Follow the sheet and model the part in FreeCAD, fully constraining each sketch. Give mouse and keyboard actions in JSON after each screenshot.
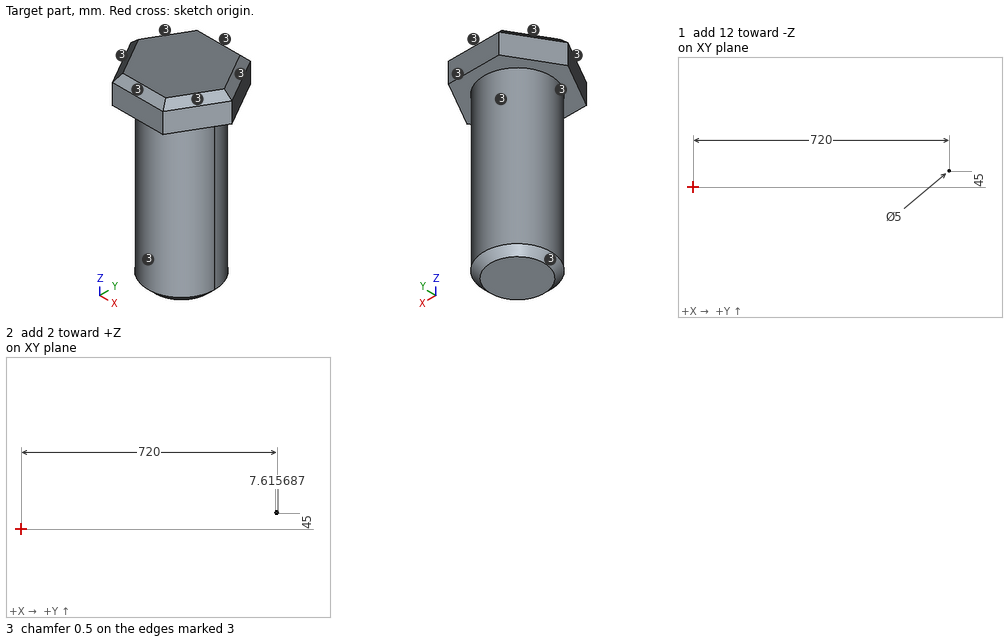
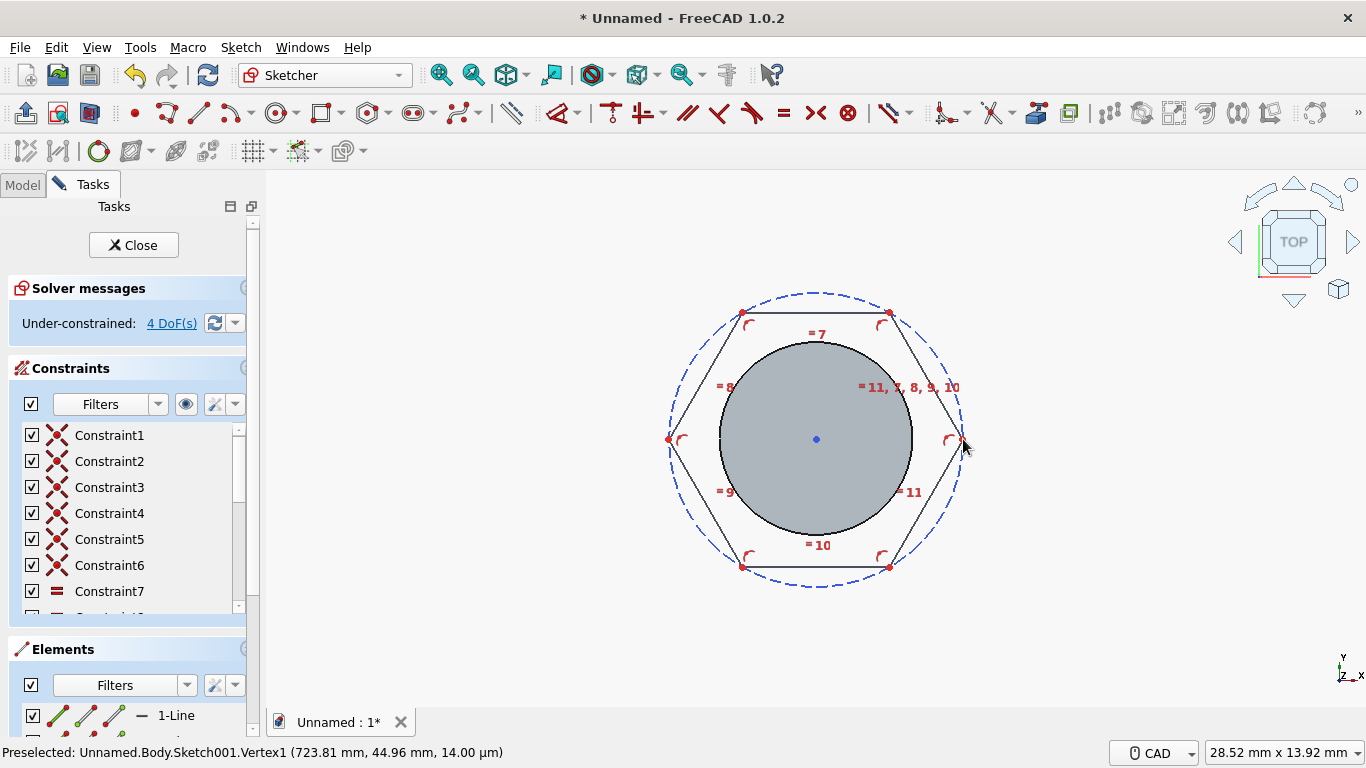
{"action": "left_click", "coordinate": [845, 313]}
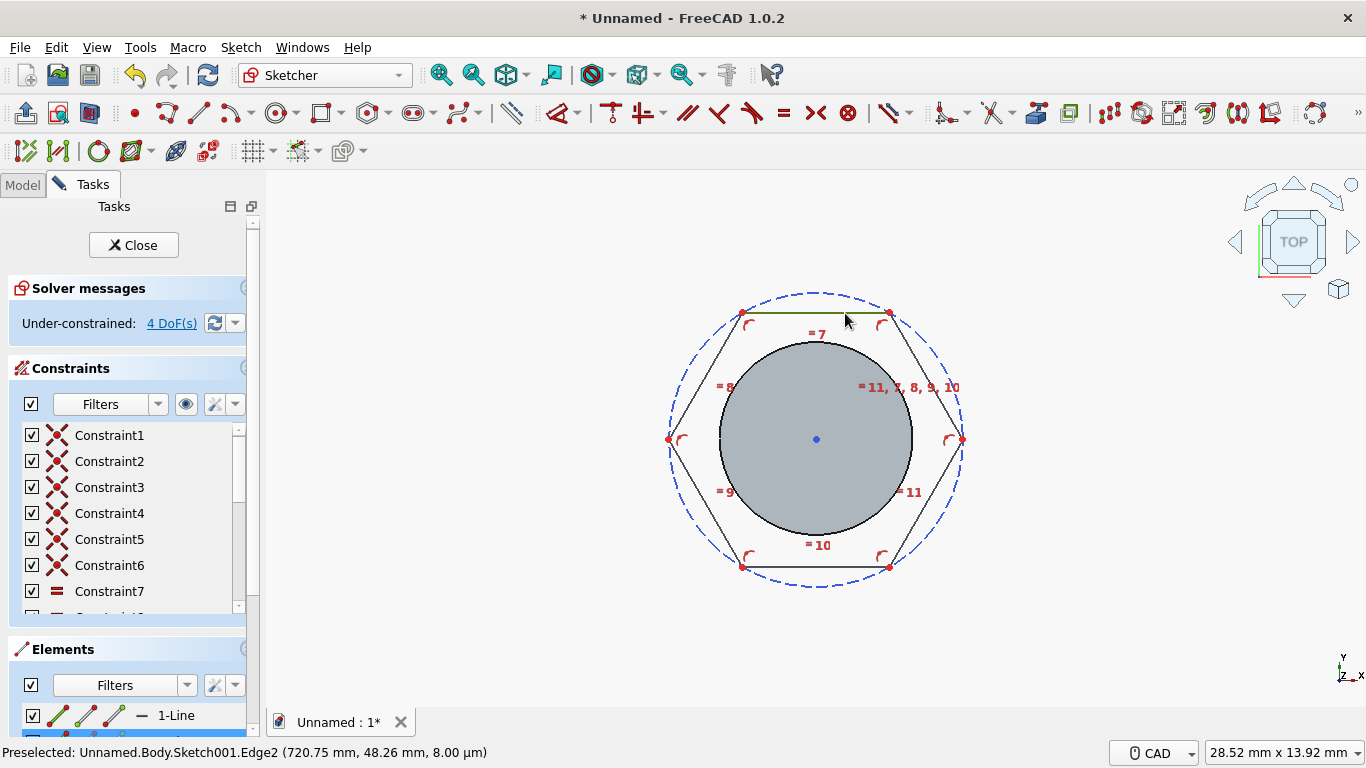
{"action": "key", "text": "h"}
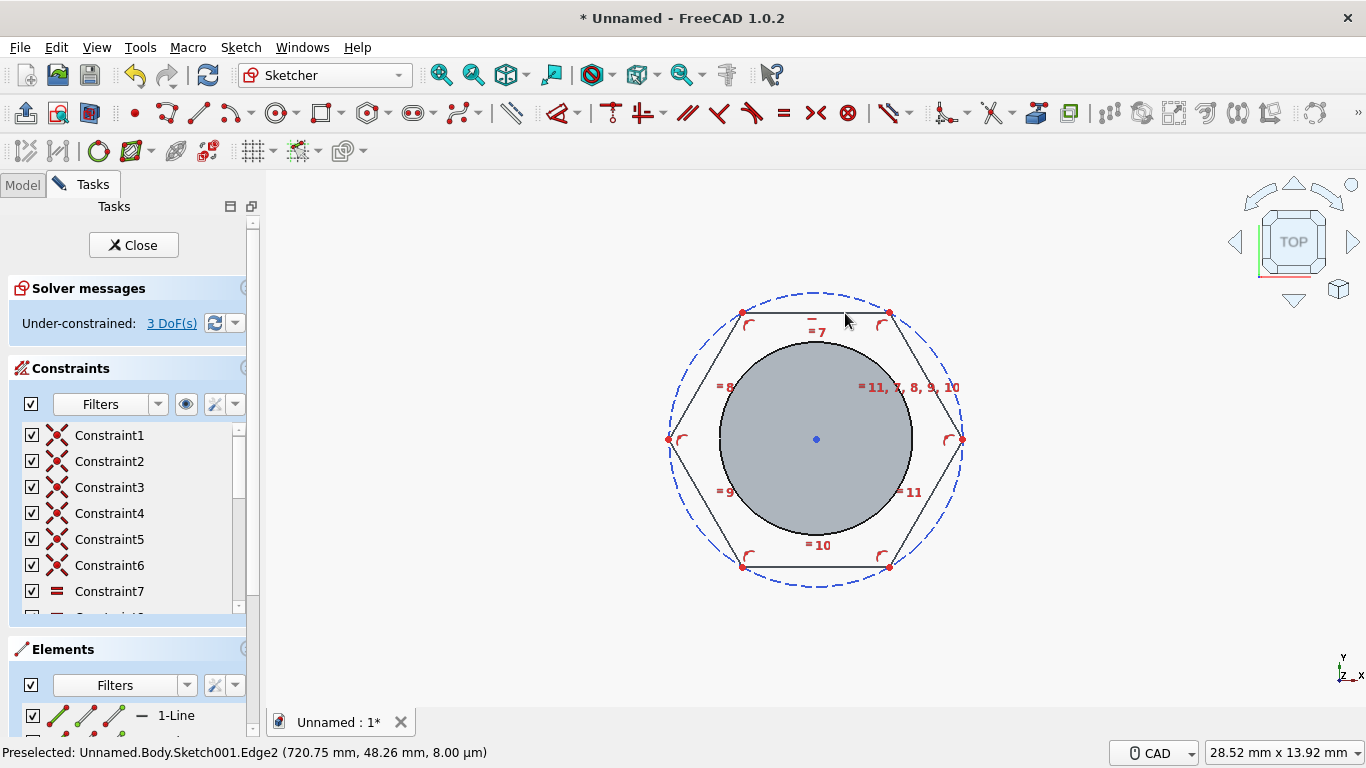
{"action": "left_click", "coordinate": [558, 114]}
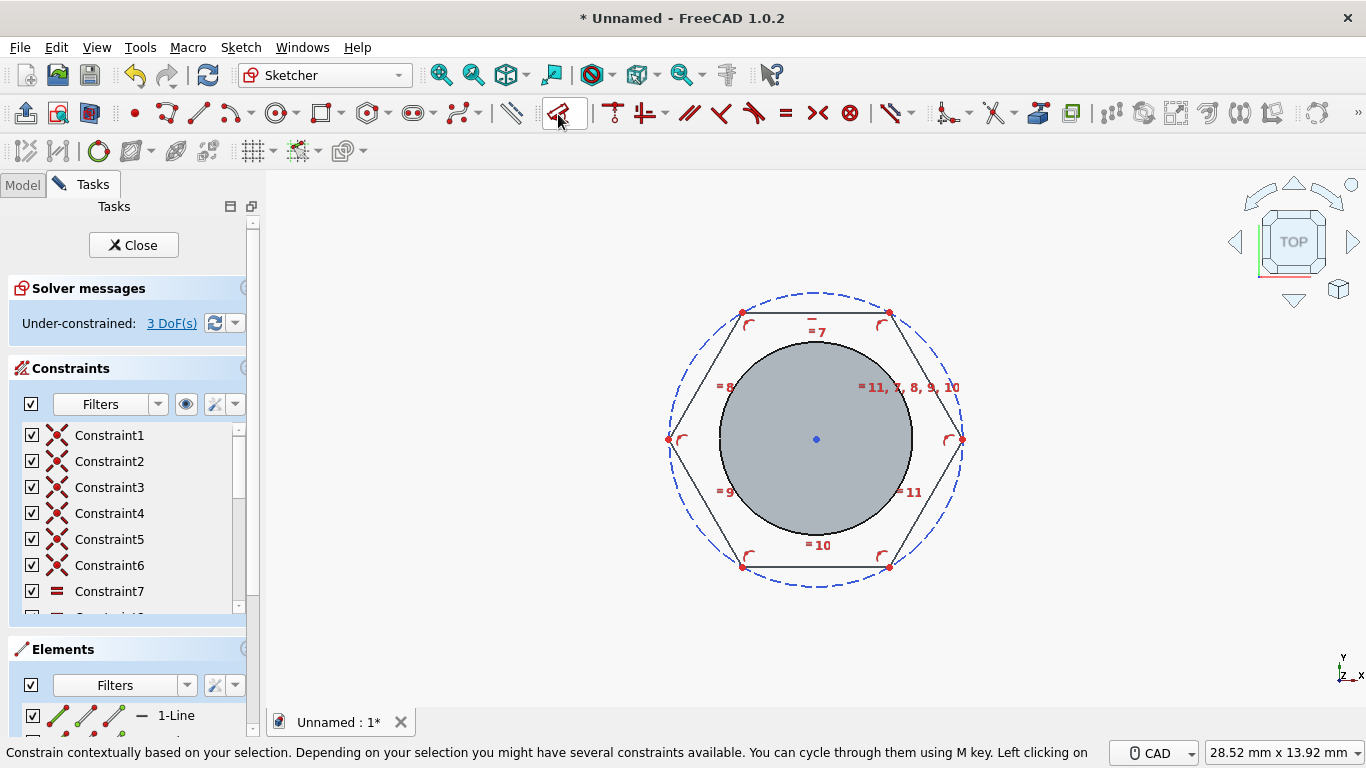
{"action": "left_click", "coordinate": [816, 440]}
{"action": "left_click", "coordinate": [850, 505]}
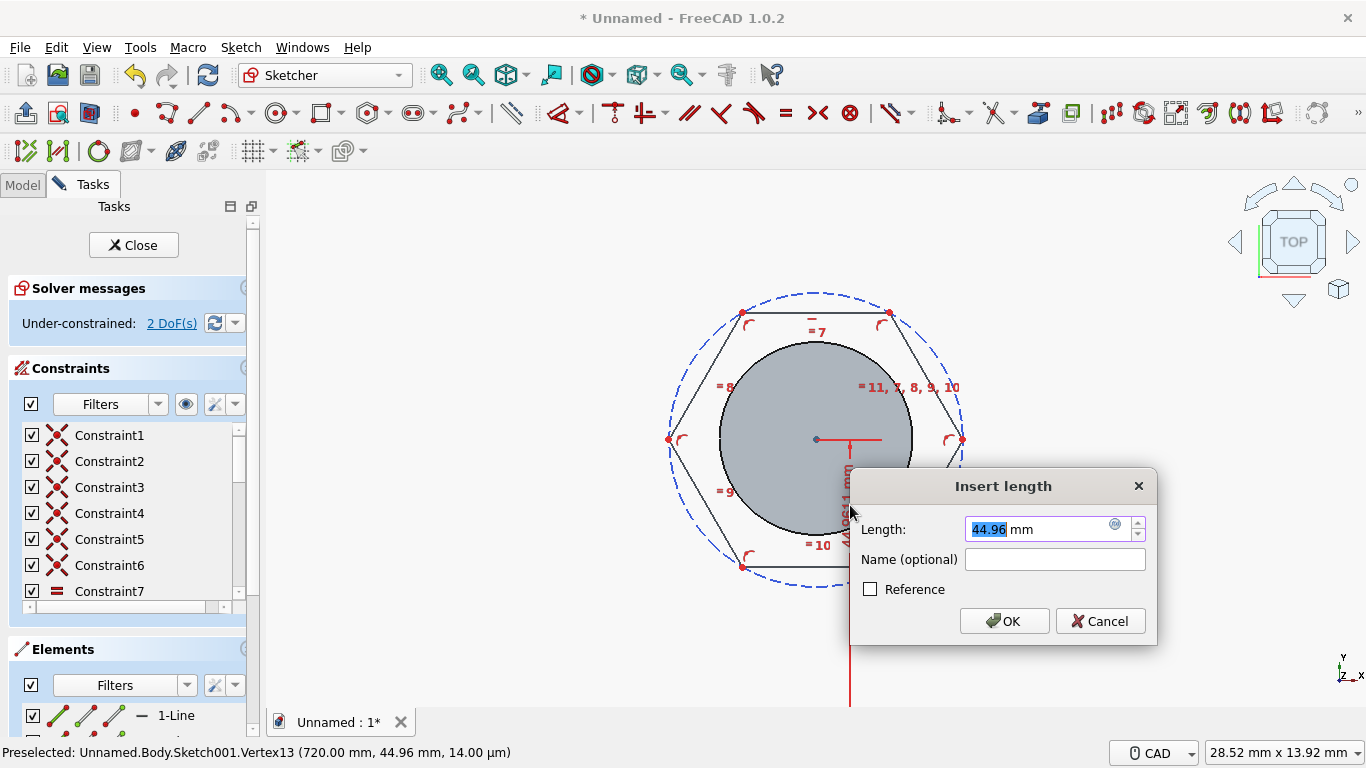
{"action": "type", "text": "45"}
{"action": "key", "text": "Return"}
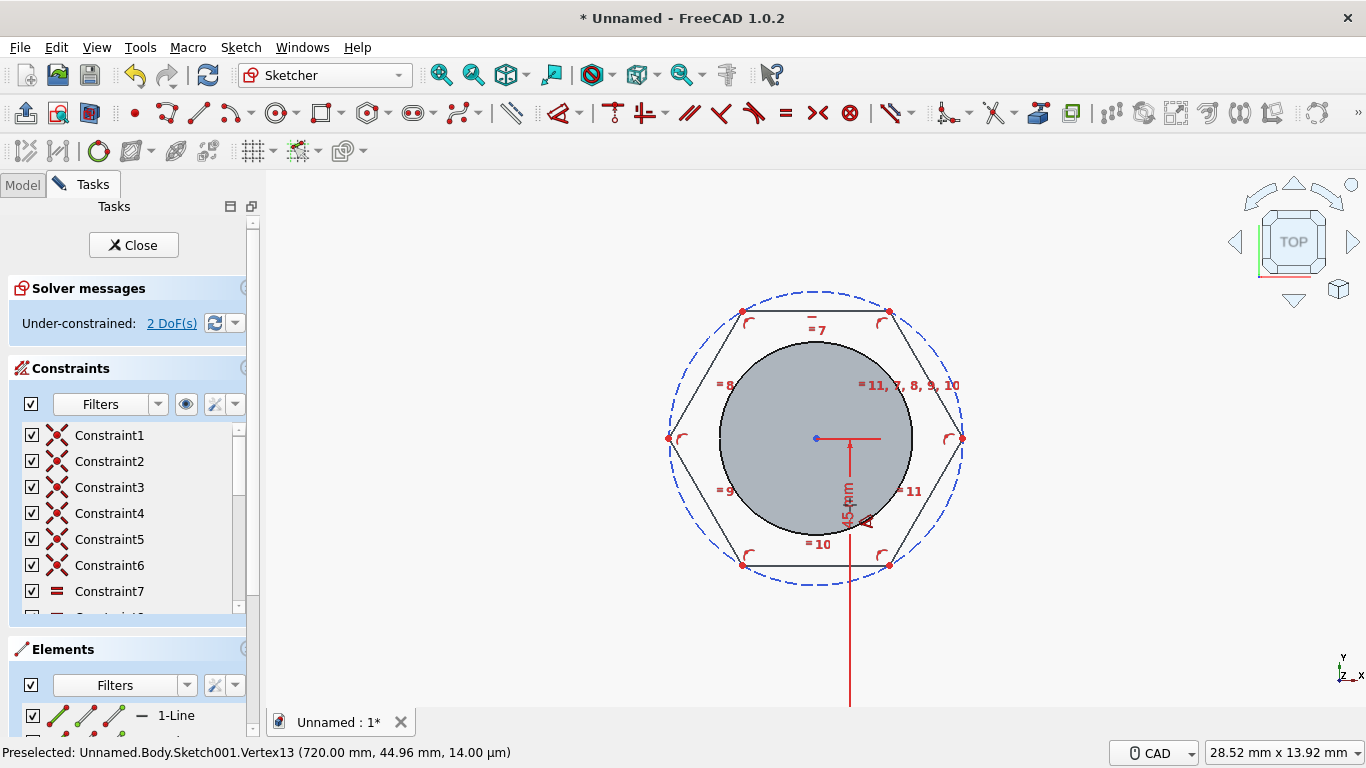
{"action": "left_click", "coordinate": [816, 439]}
{"action": "left_click", "coordinate": [555, 405]}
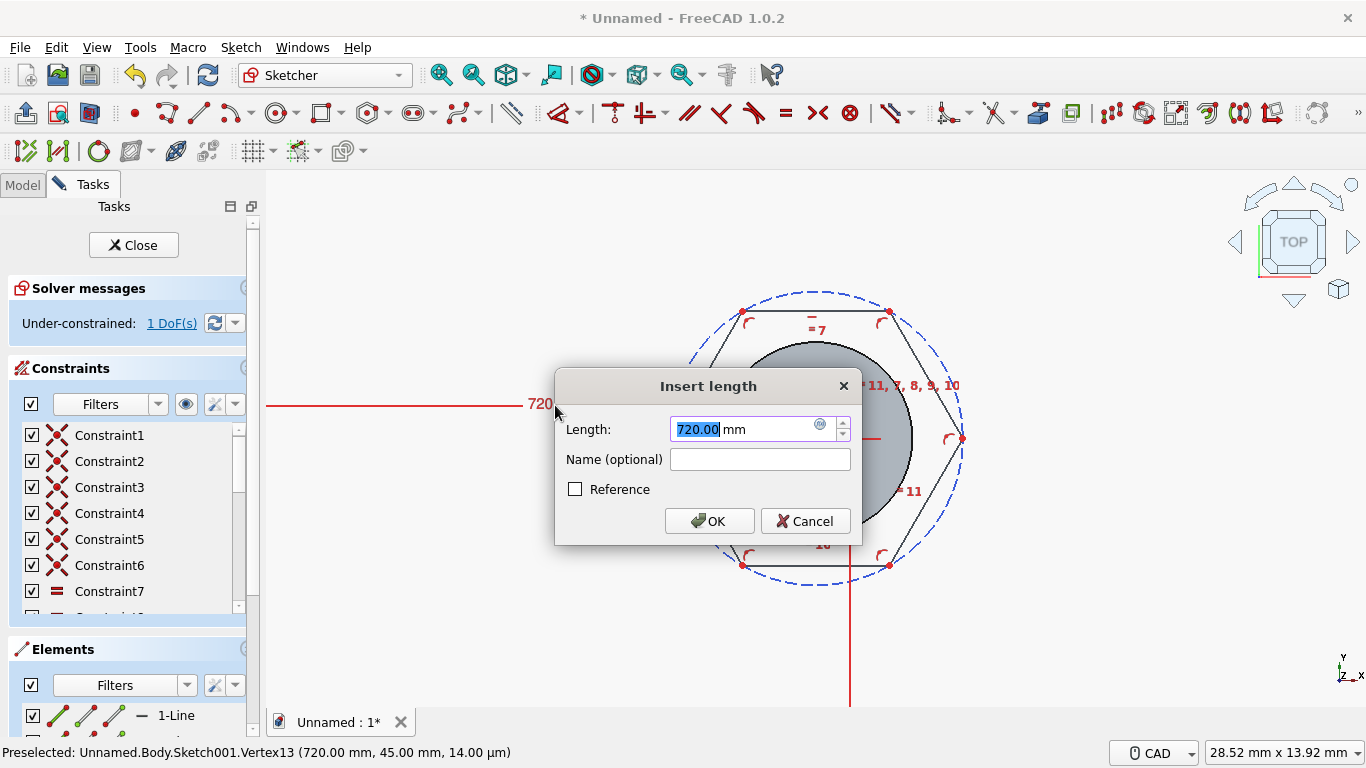
{"action": "type", "text": "720"}
{"action": "key", "text": "Return"}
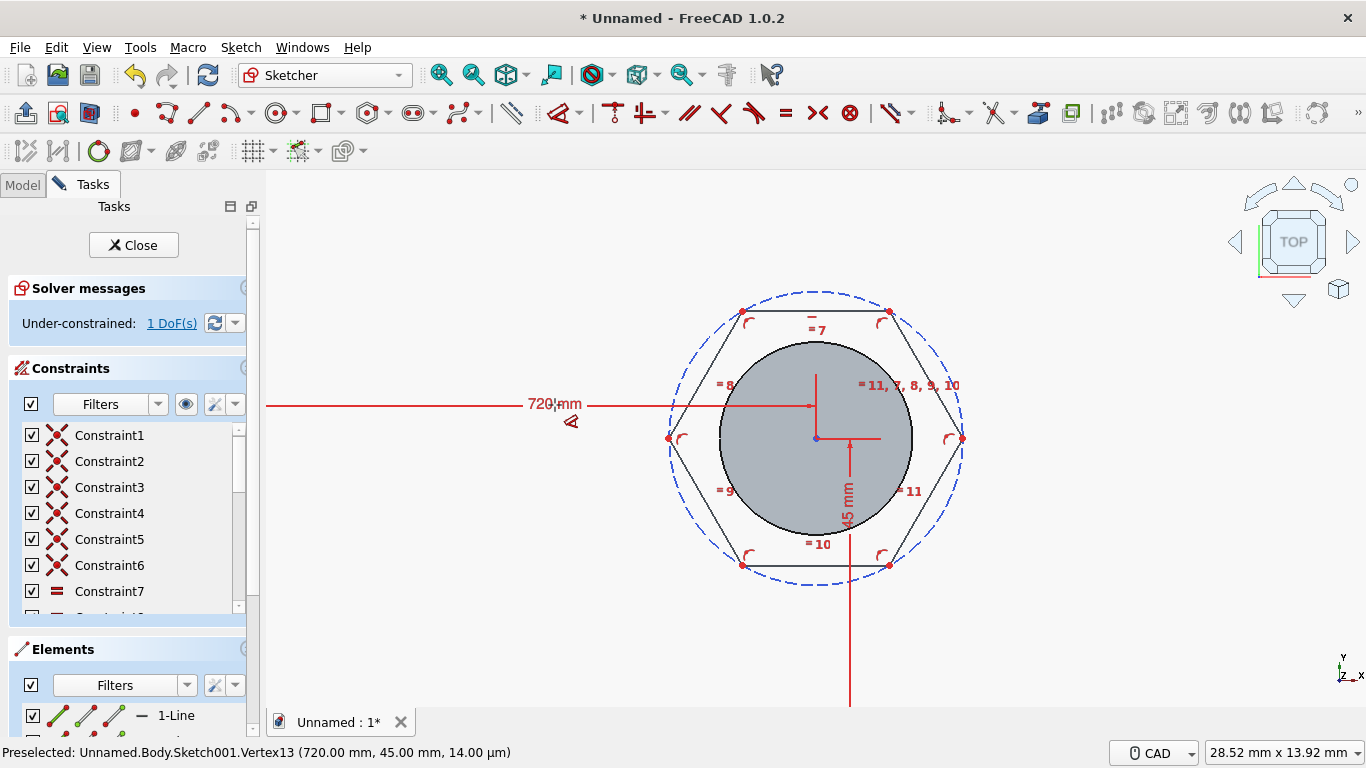
{"action": "left_click", "coordinate": [669, 438]}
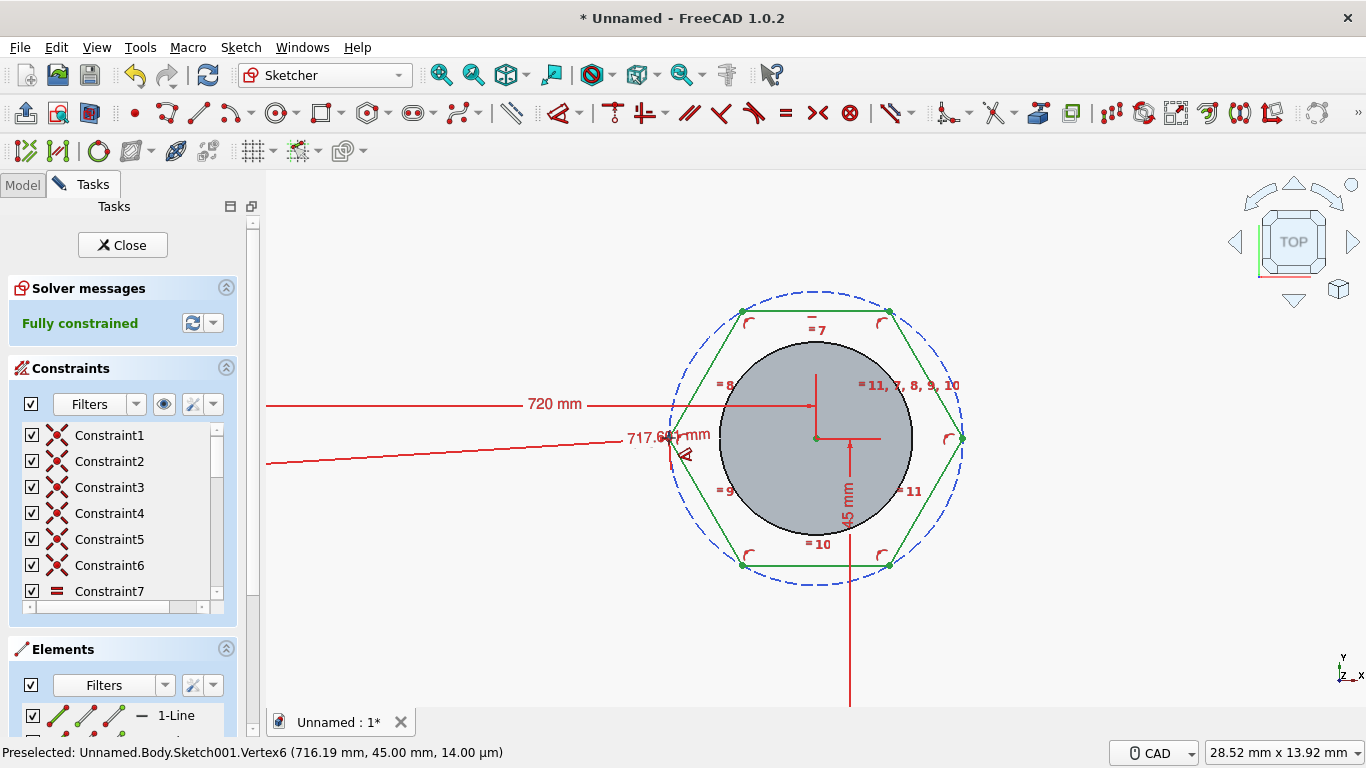
{"action": "left_click", "coordinate": [963, 439]}
{"action": "left_click", "coordinate": [816, 404]}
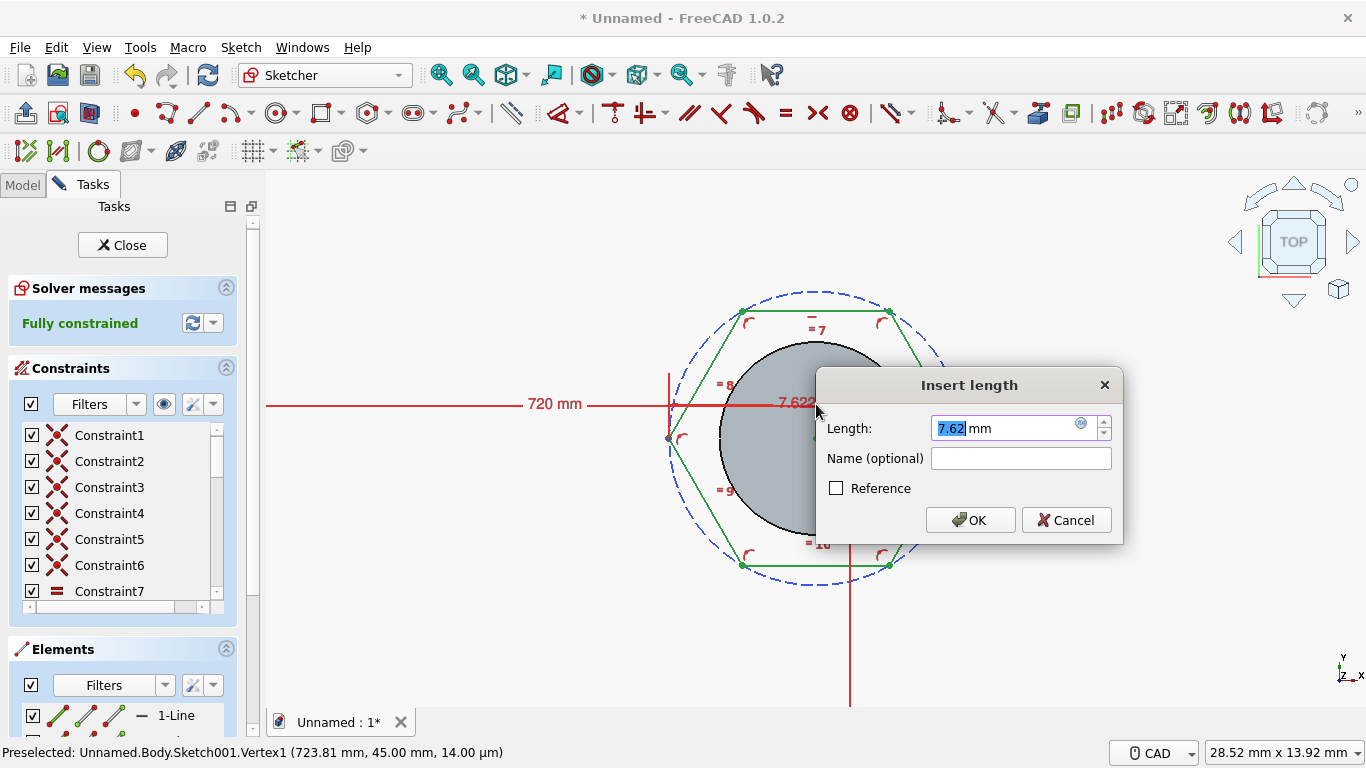
{"action": "type", "text": "7.615687"}
{"action": "key", "text": "Return"}
{"action": "key", "text": "Escape"}